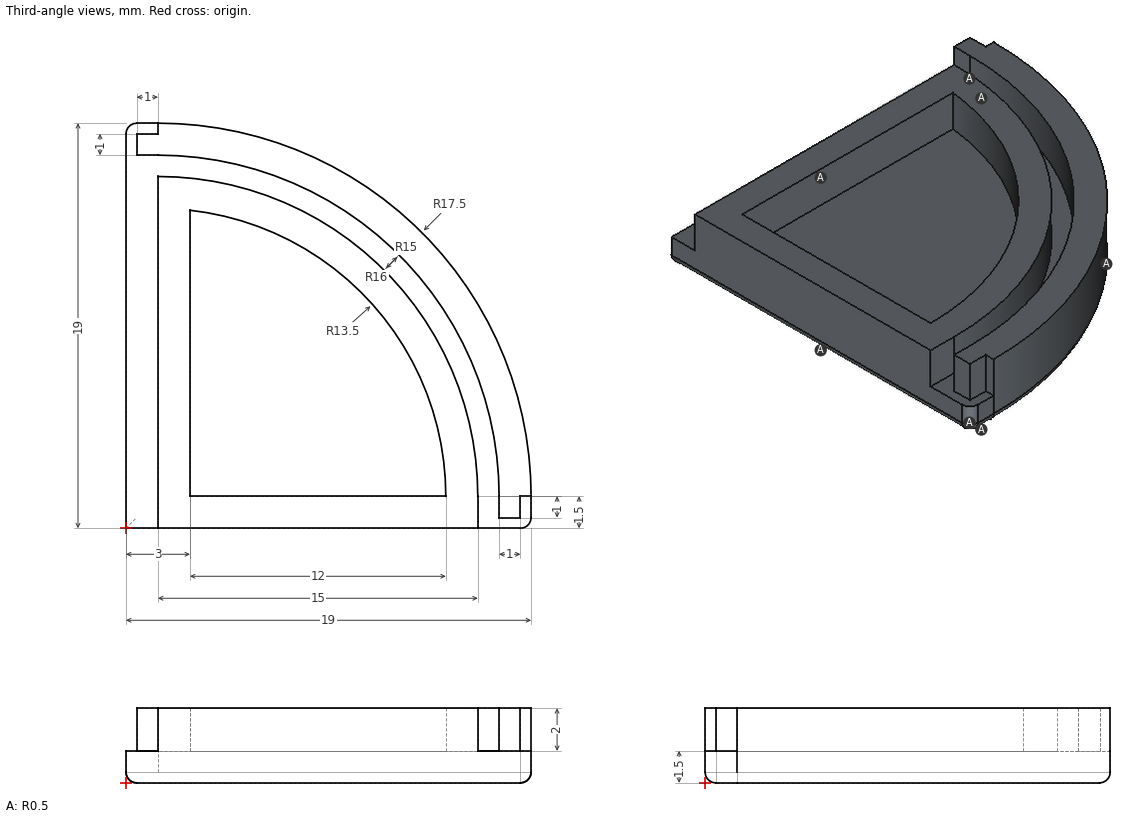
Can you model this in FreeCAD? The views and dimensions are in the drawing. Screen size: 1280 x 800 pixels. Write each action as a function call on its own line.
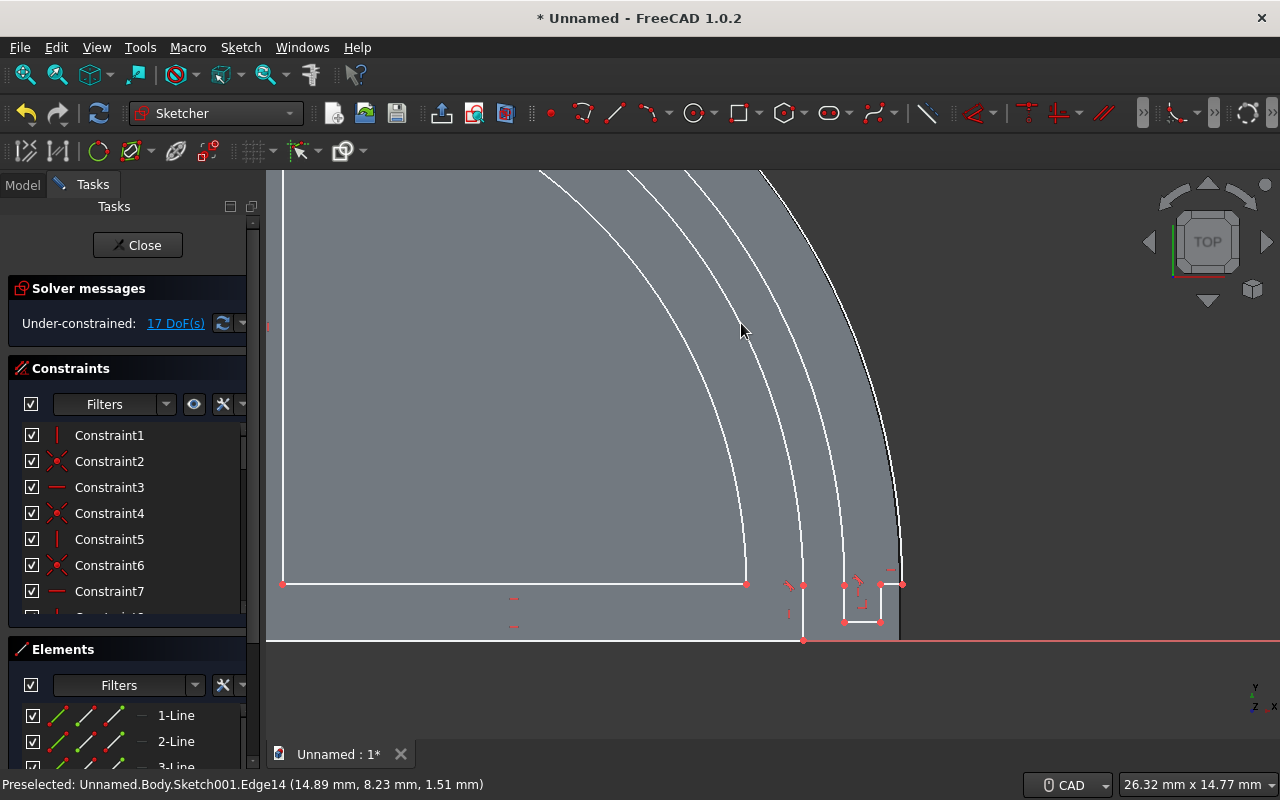
click(777, 304)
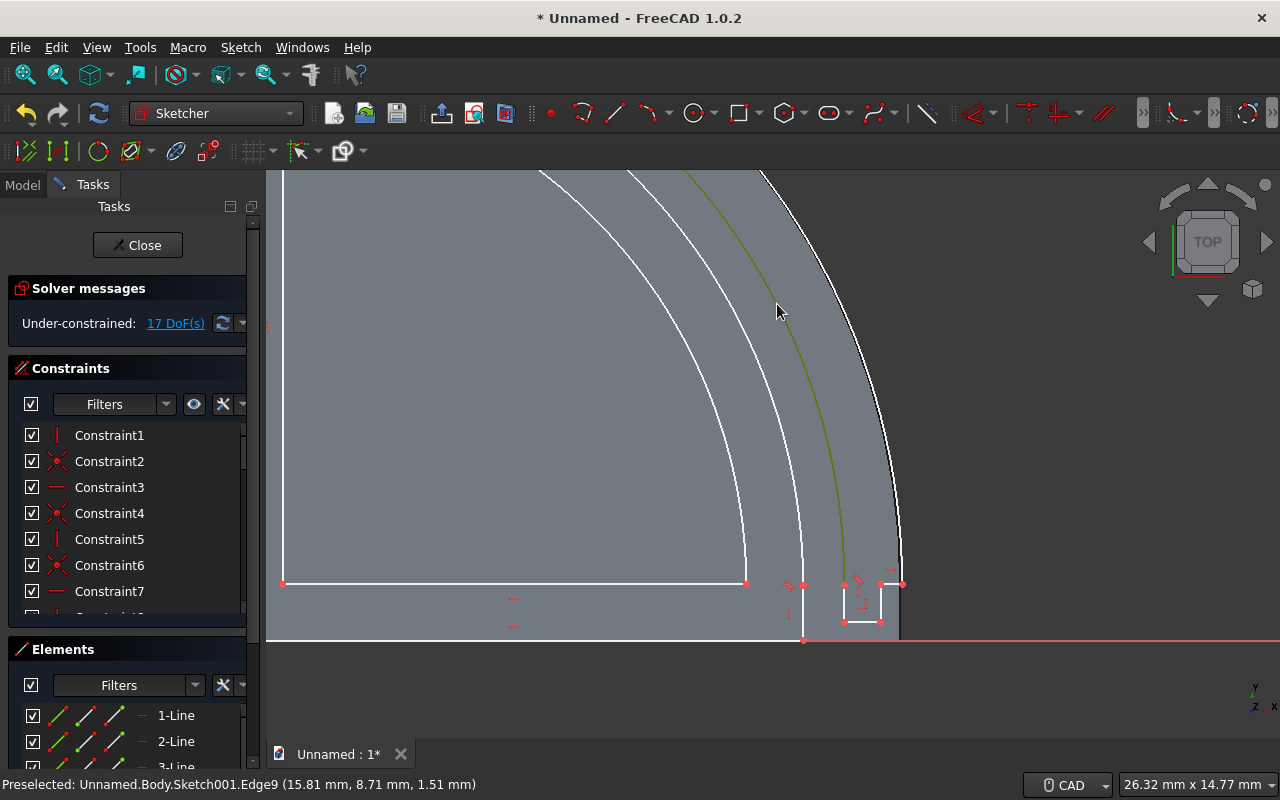
click(696, 364)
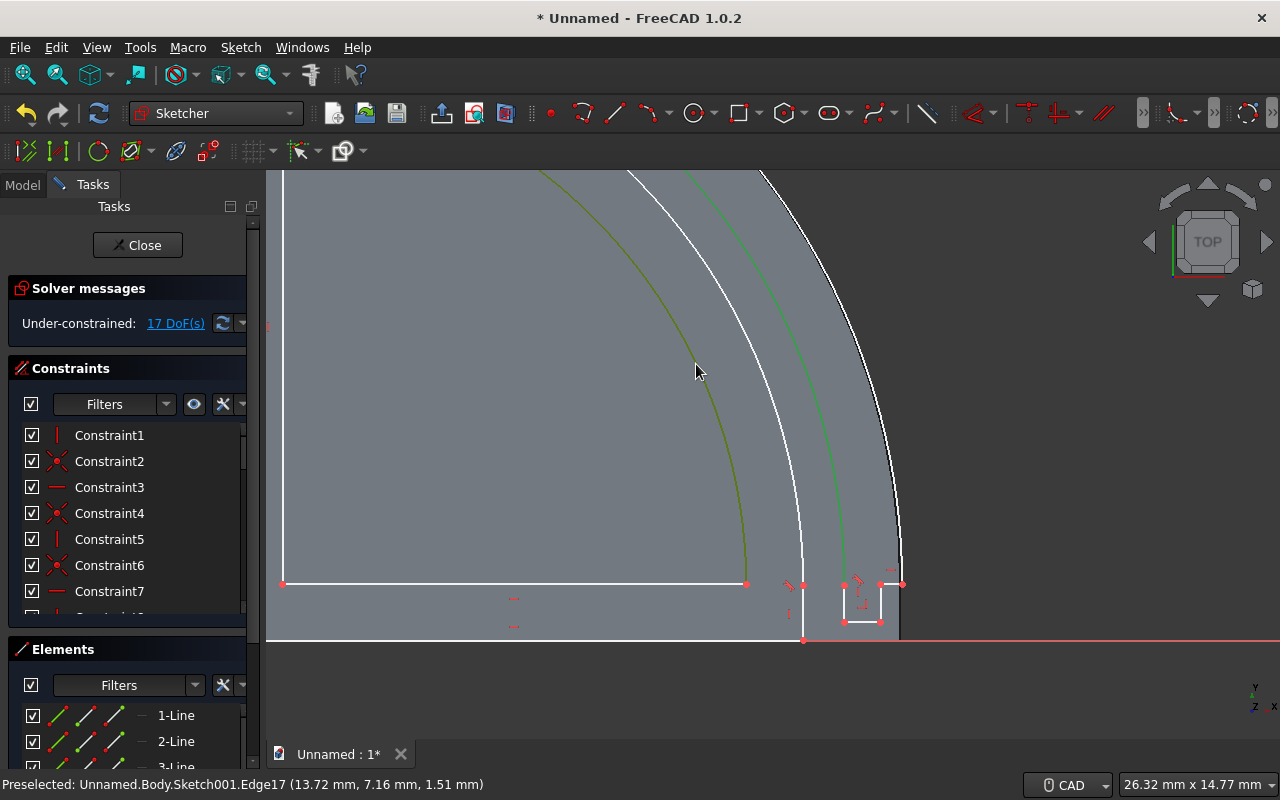
key(c)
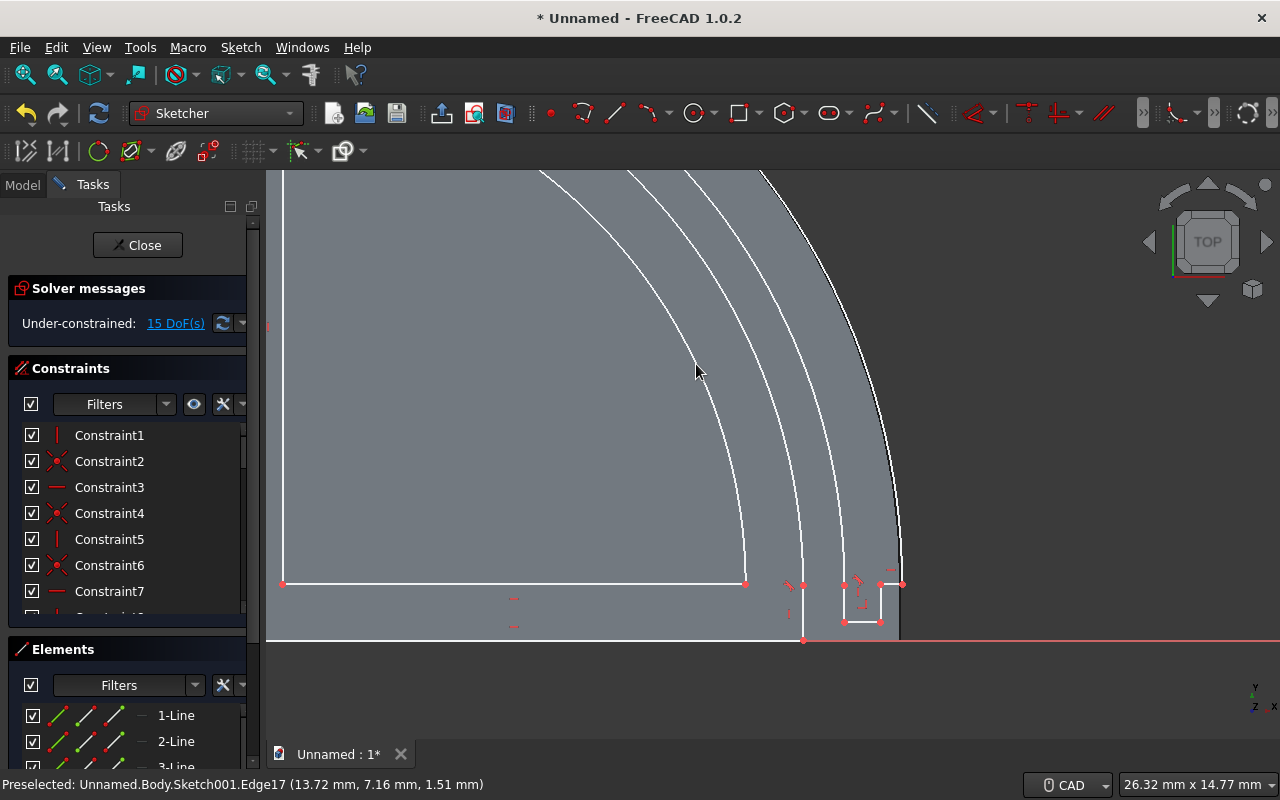
key(d)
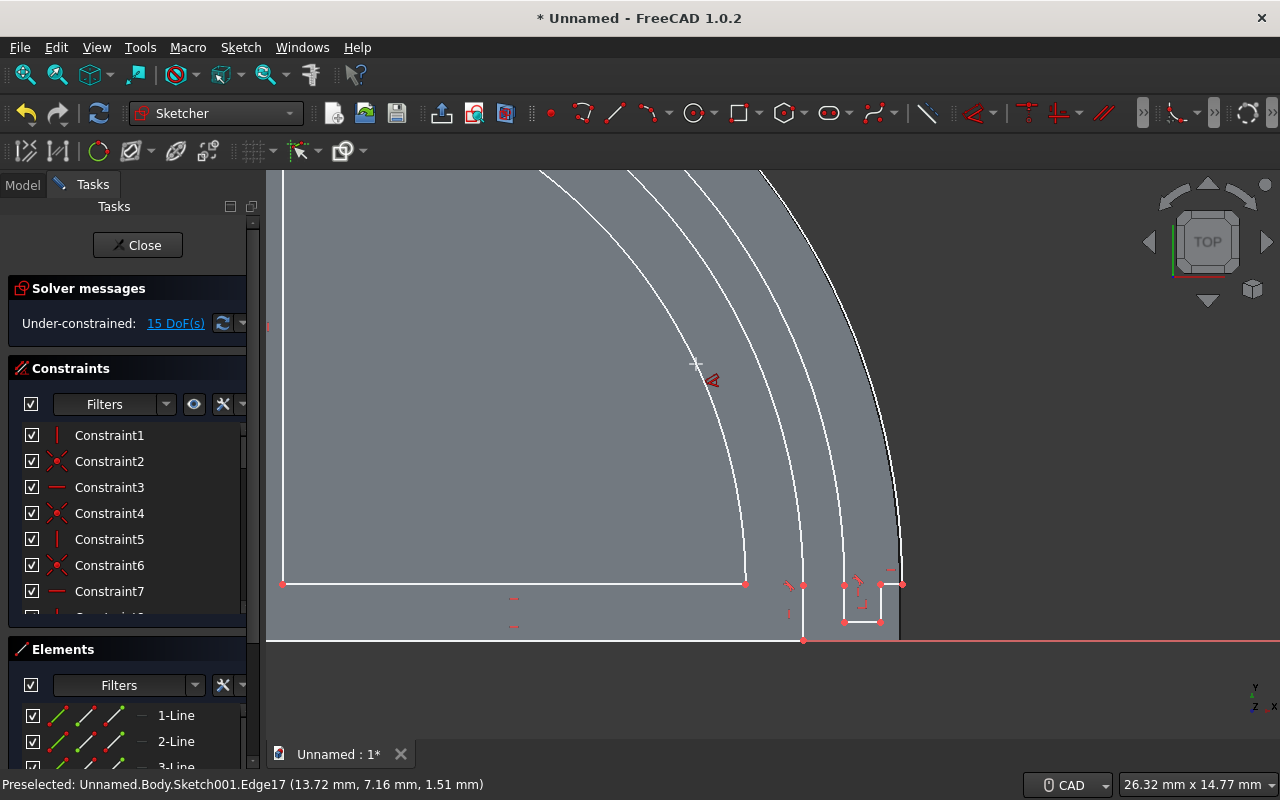
click(777, 304)
click(806, 289)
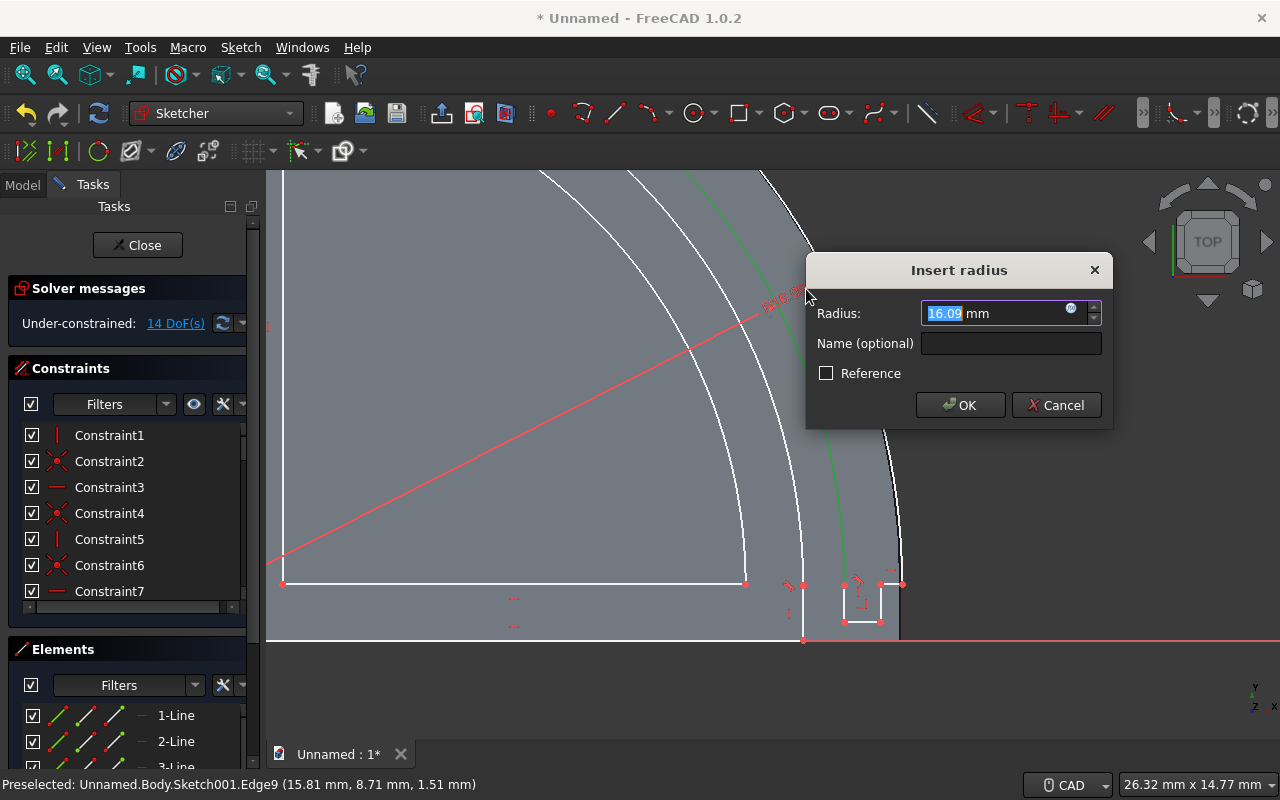
text(16)
key(Return)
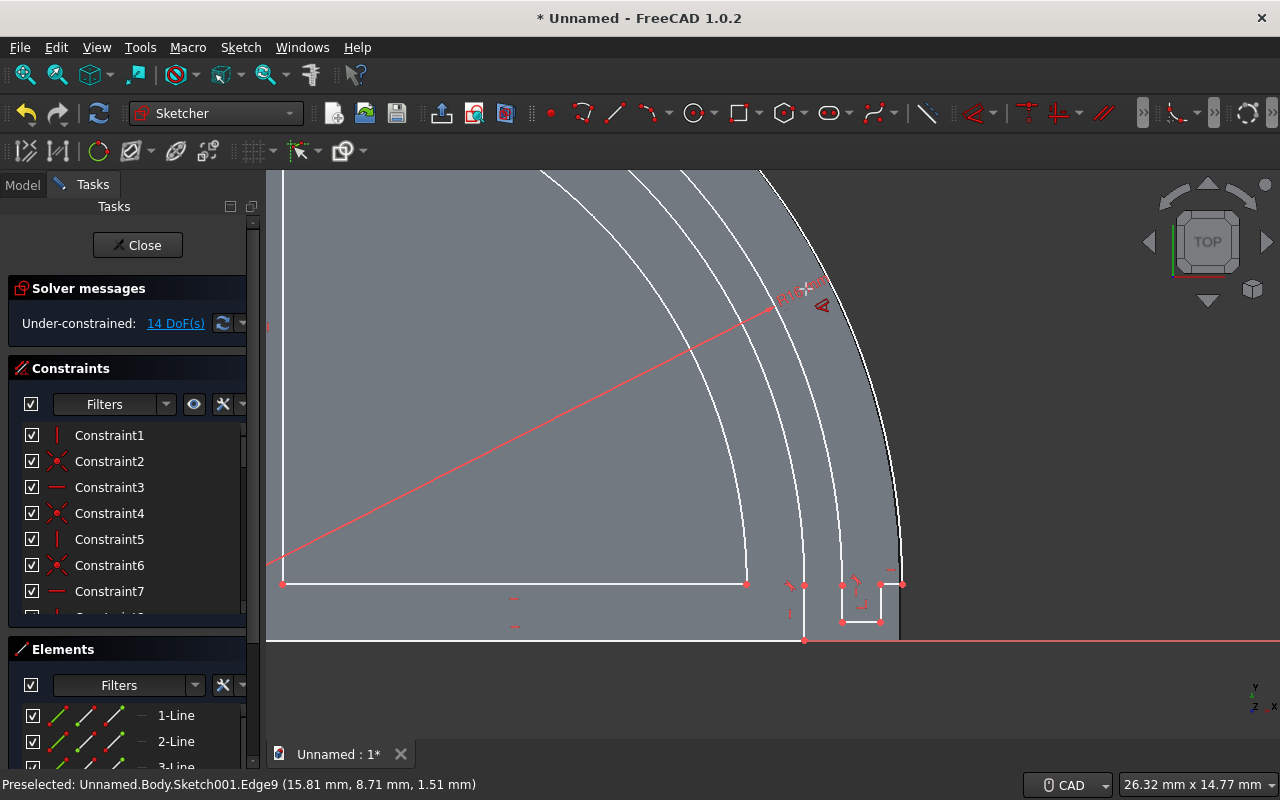
click(828, 278)
click(856, 263)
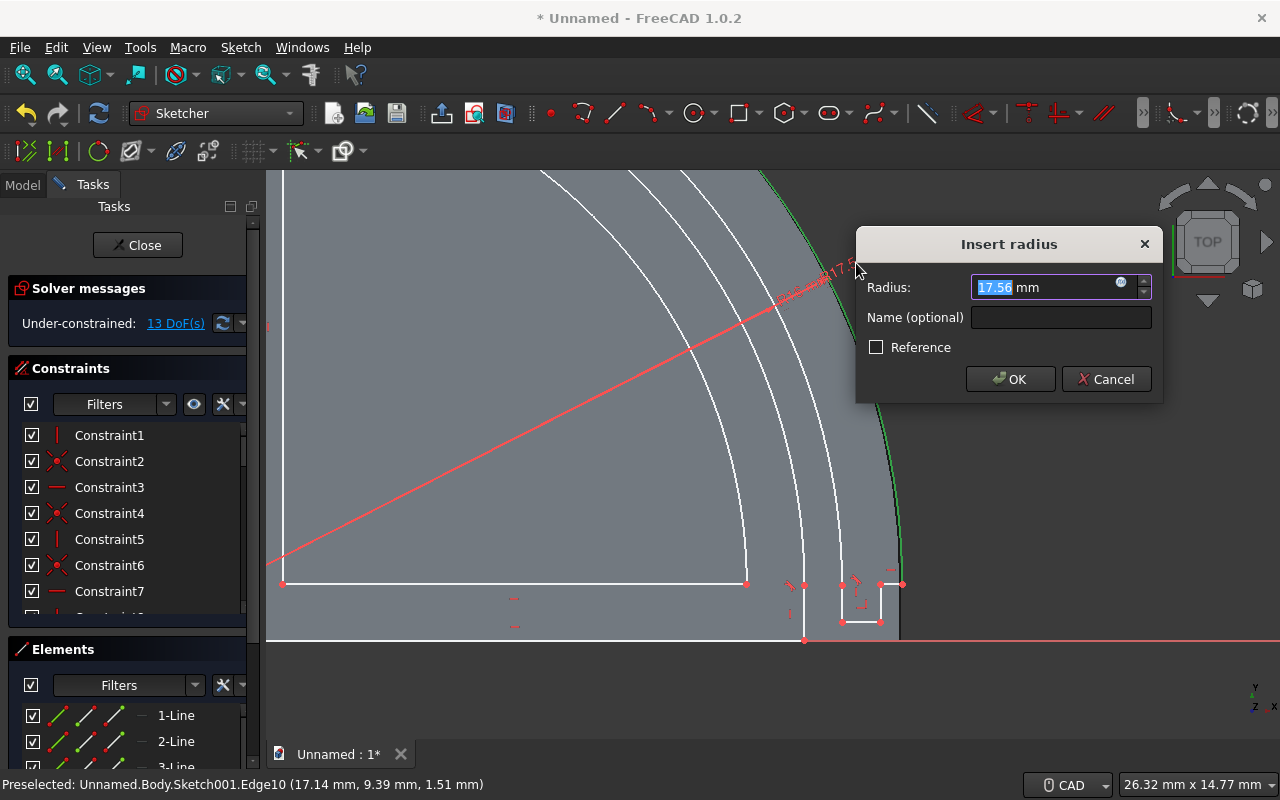
text(17.5)
key(Return)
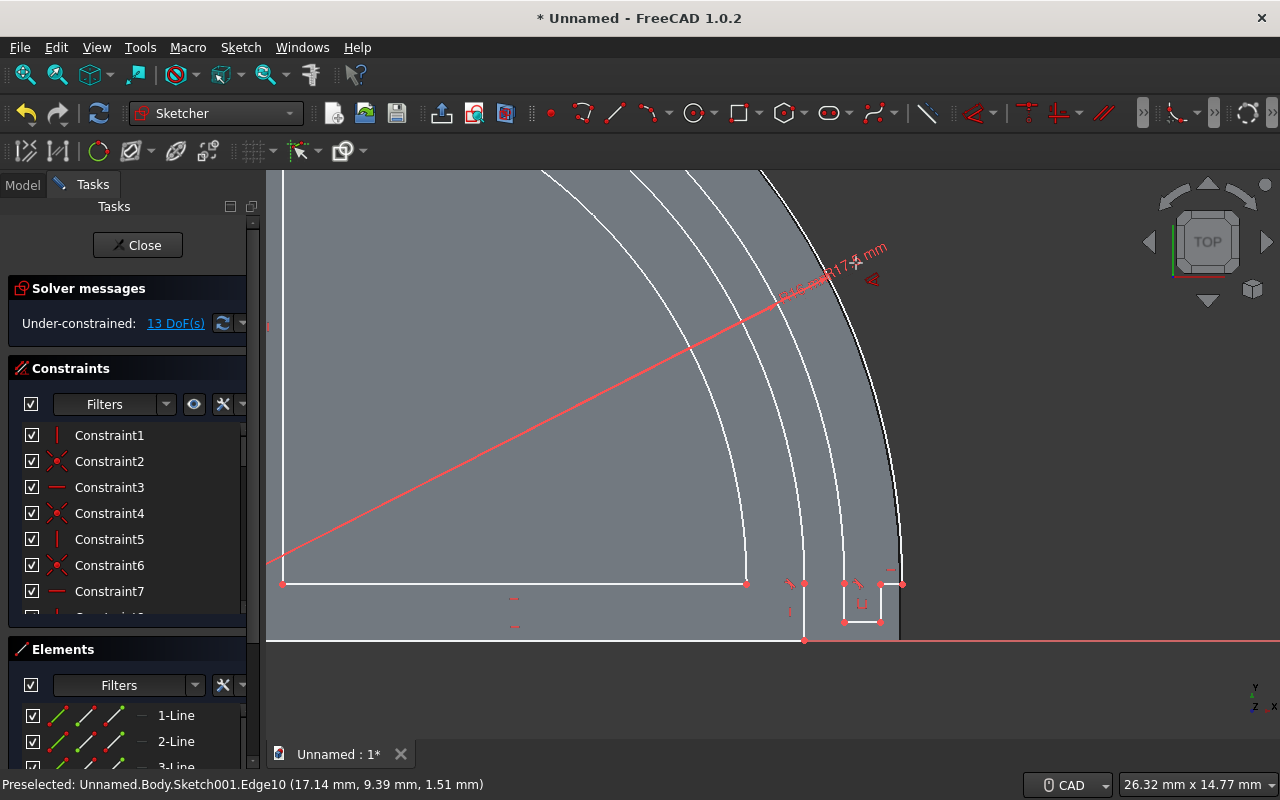
click(741, 321)
click(859, 601)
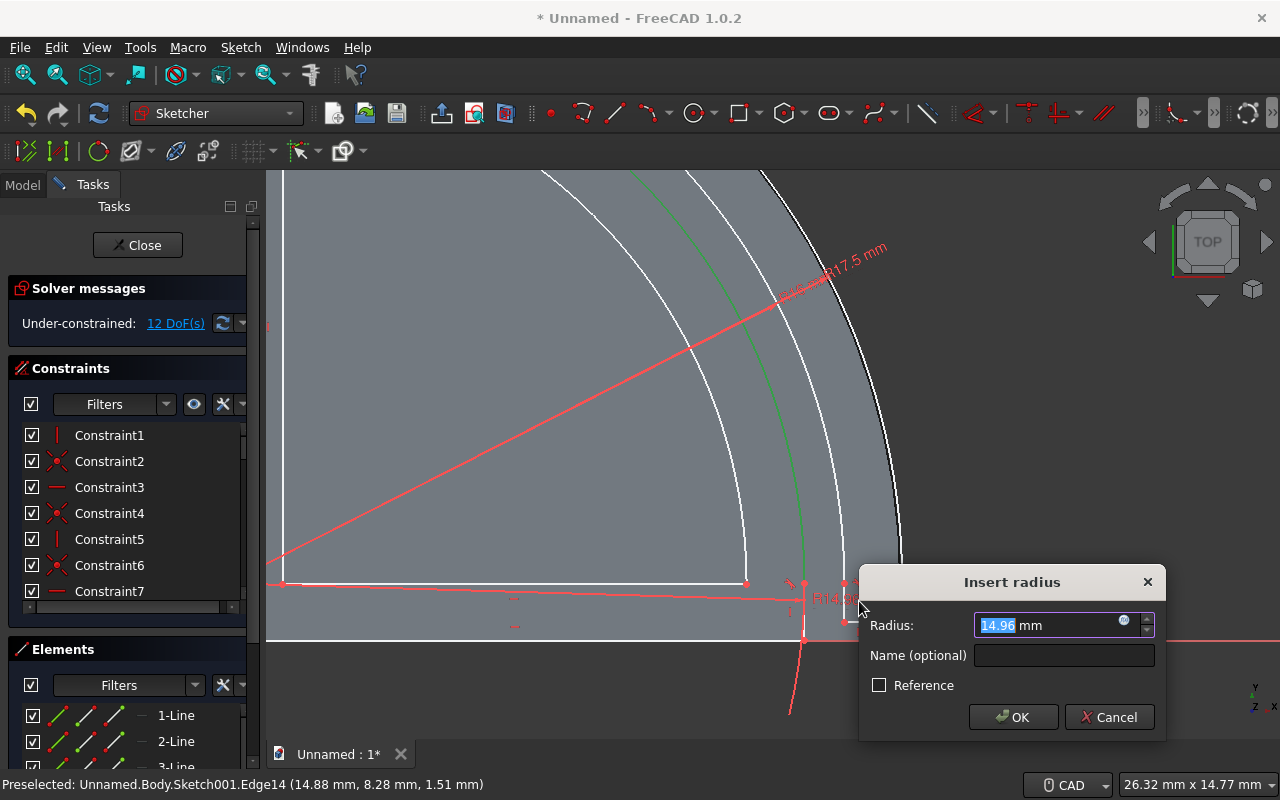
text(15)
key(Return)